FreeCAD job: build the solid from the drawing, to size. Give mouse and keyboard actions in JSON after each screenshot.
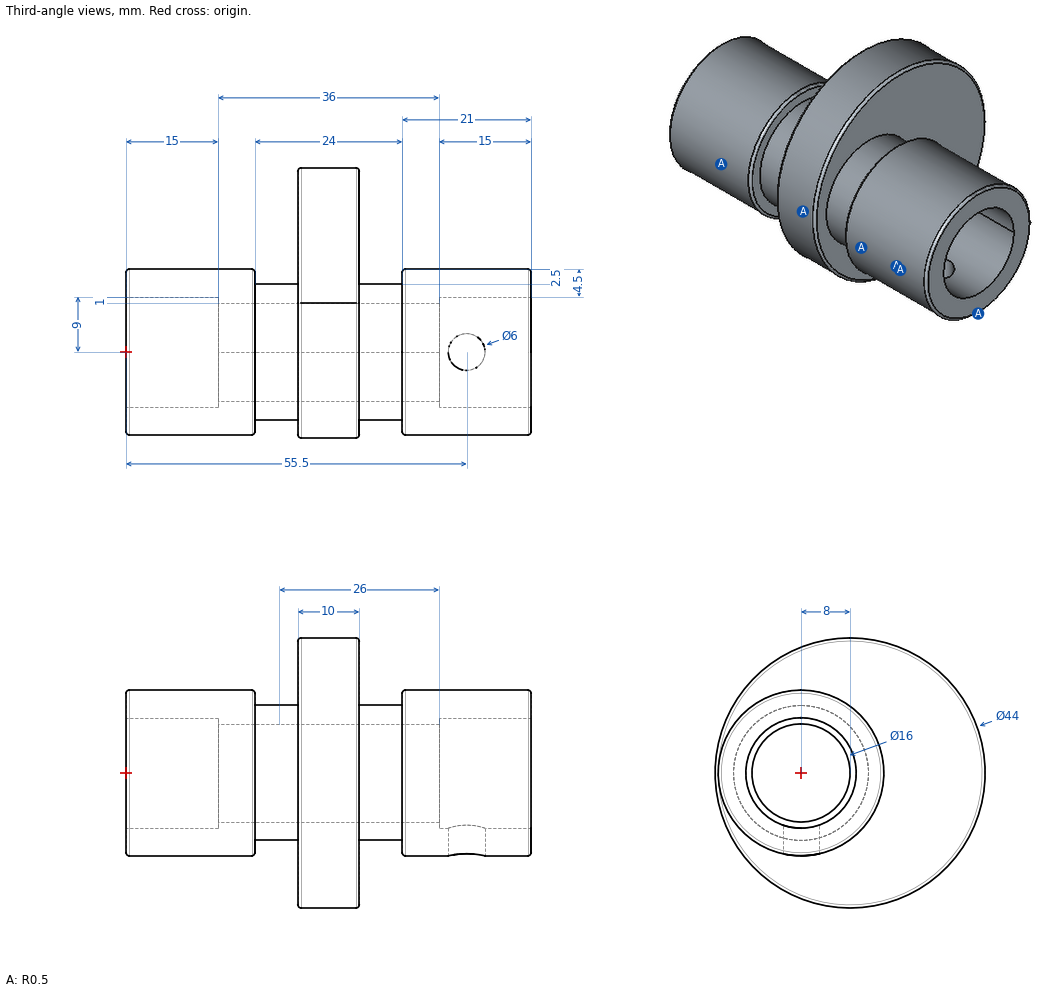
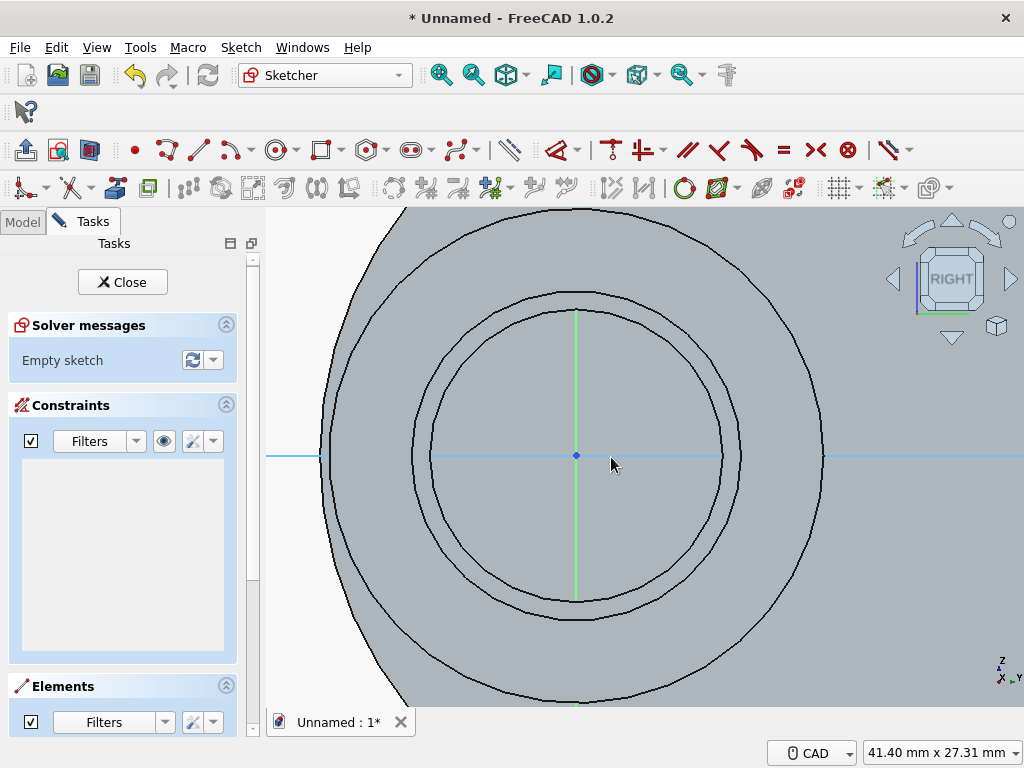
{"action": "left_click", "coordinate": [276, 150]}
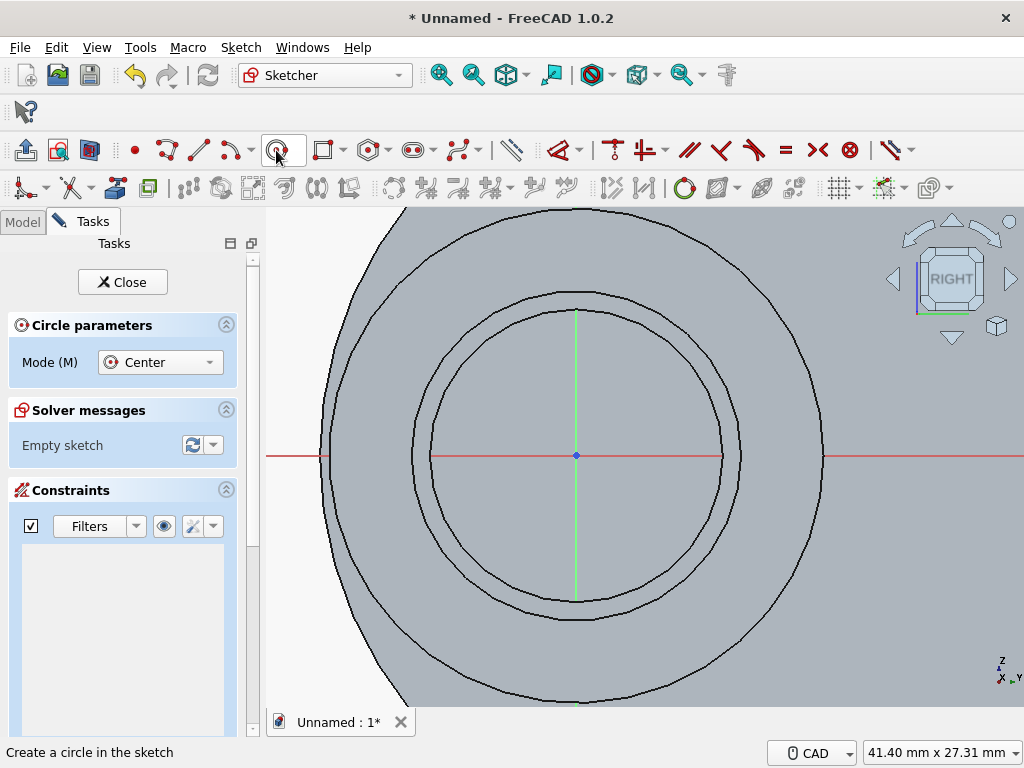
{"action": "left_click", "coordinate": [576, 456]}
{"action": "mouse_move", "coordinate": [680, 352]}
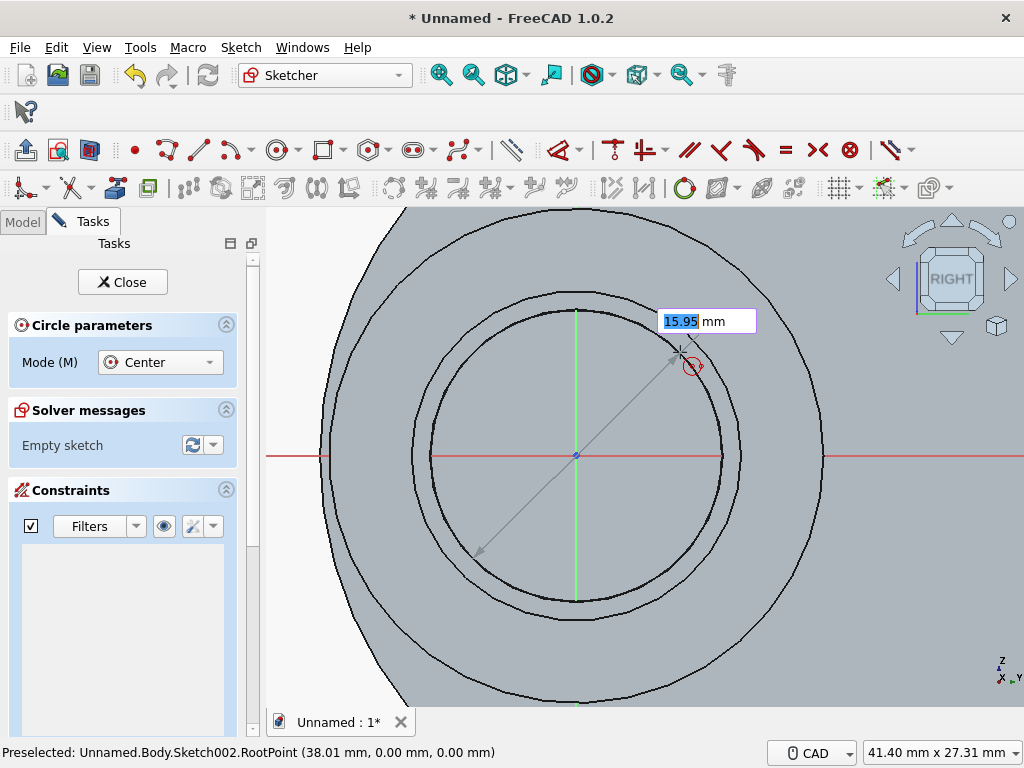
{"action": "type", "text": "16"}
{"action": "key", "text": "Return"}
{"action": "key", "text": "Escape"}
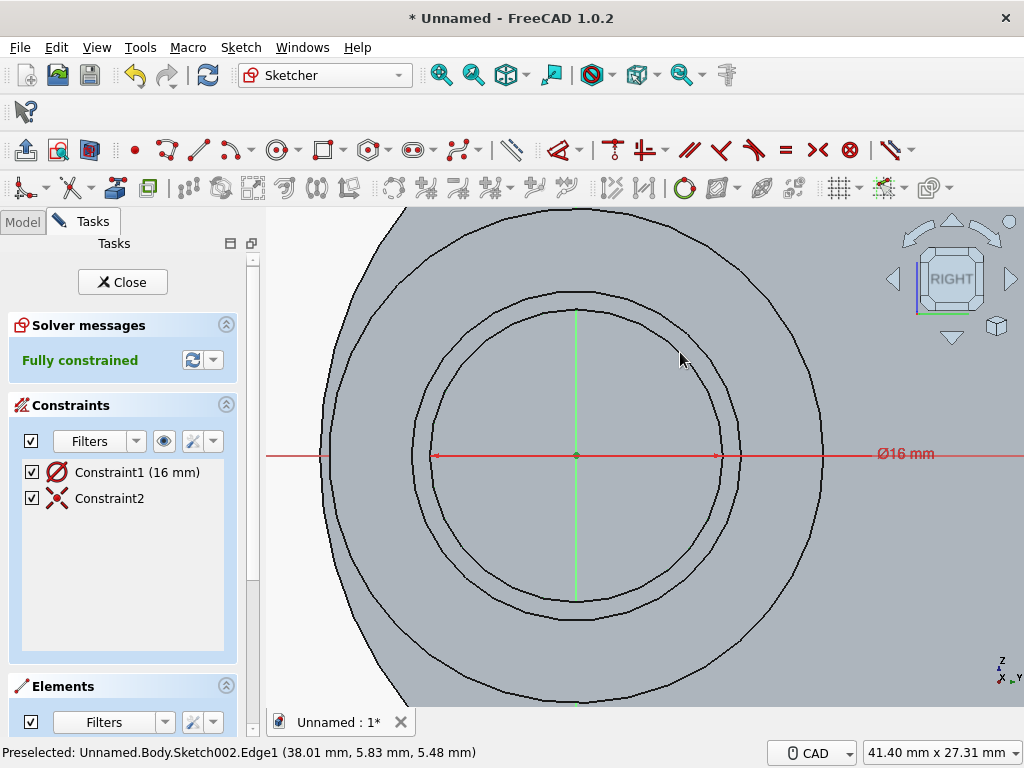
{"action": "left_click", "coordinate": [123, 282]}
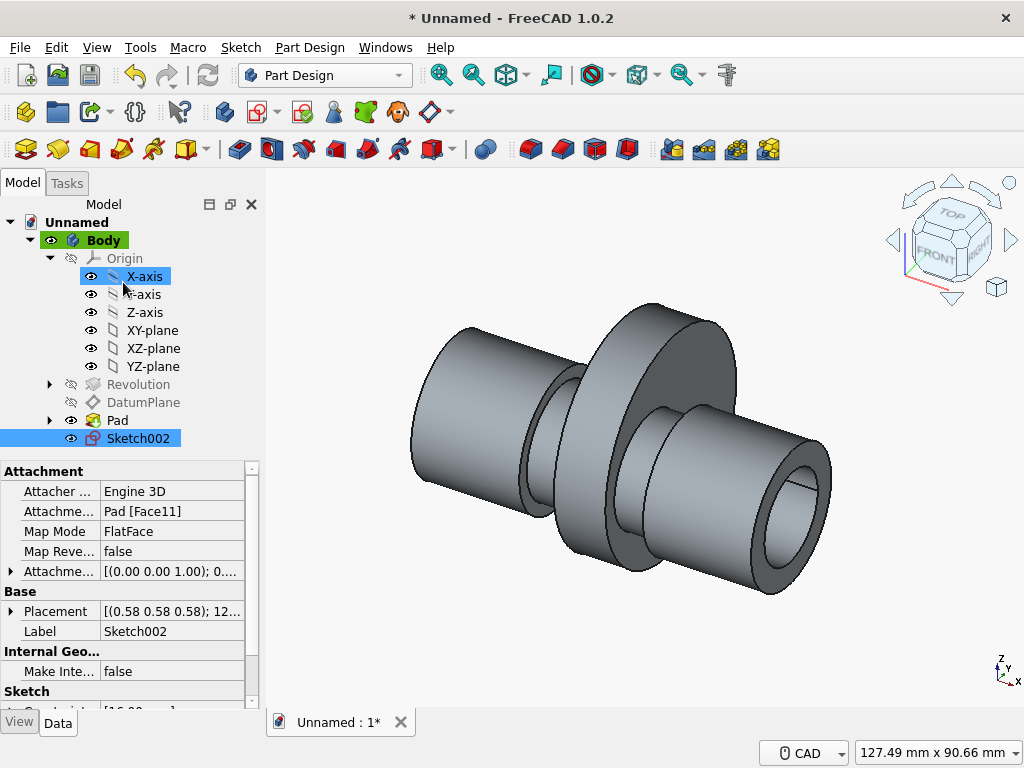
{"action": "left_click", "coordinate": [240, 150]}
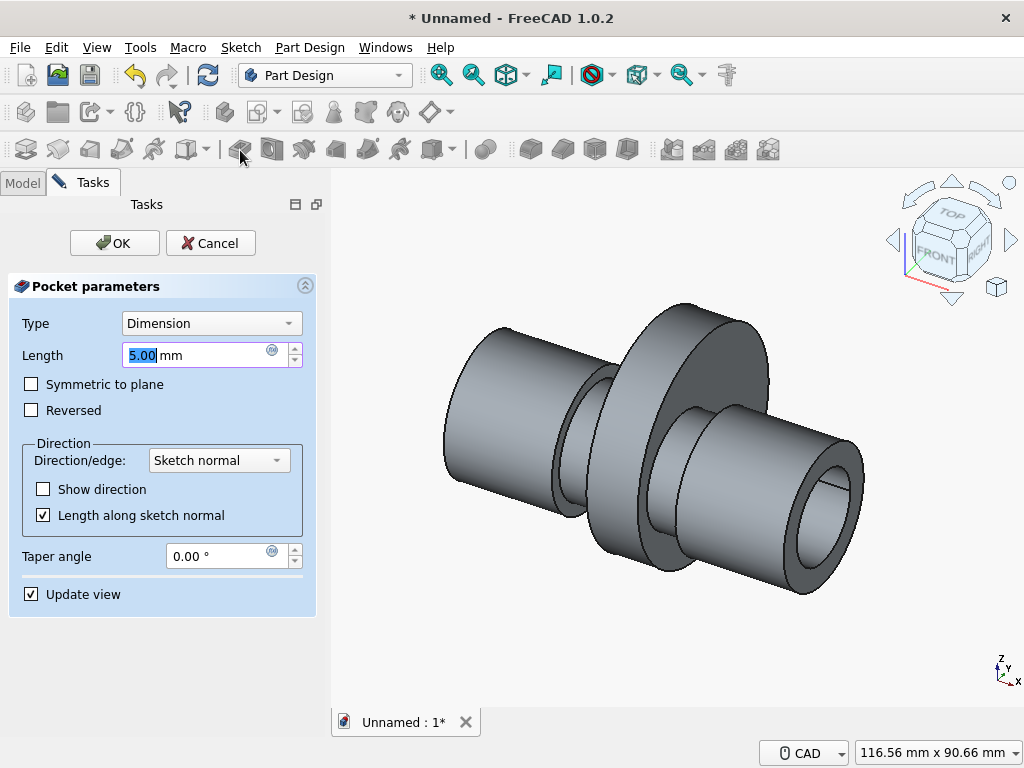
{"action": "type", "text": "26"}
{"action": "key", "text": "Tab"}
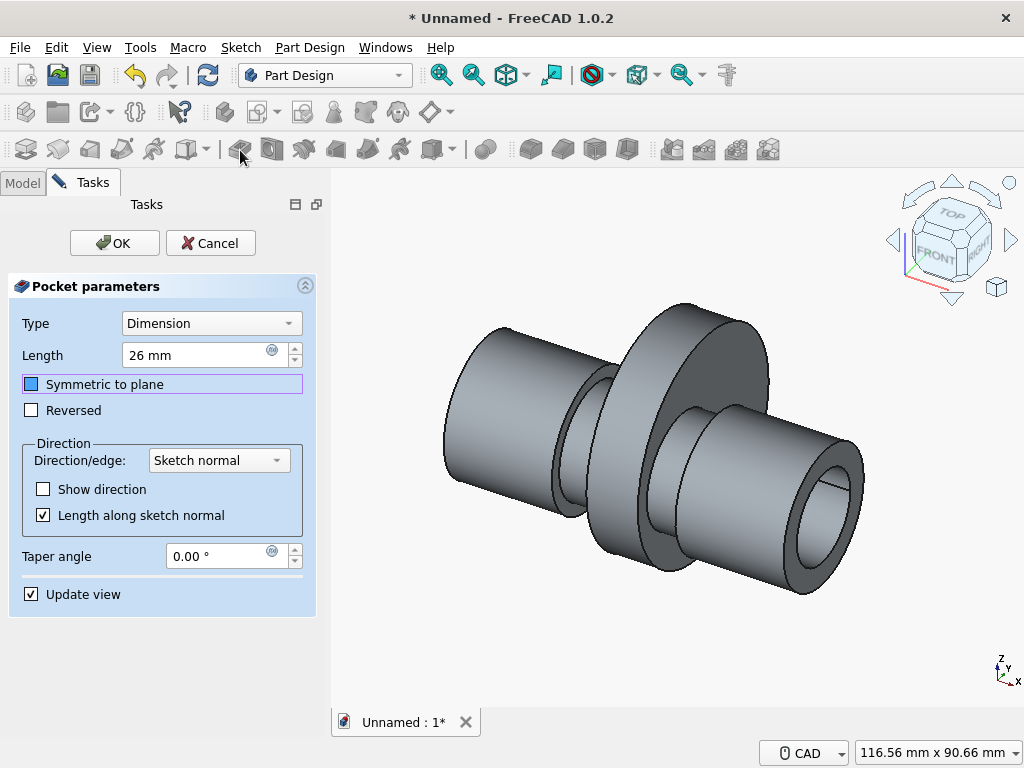
{"action": "left_click", "coordinate": [30, 384]}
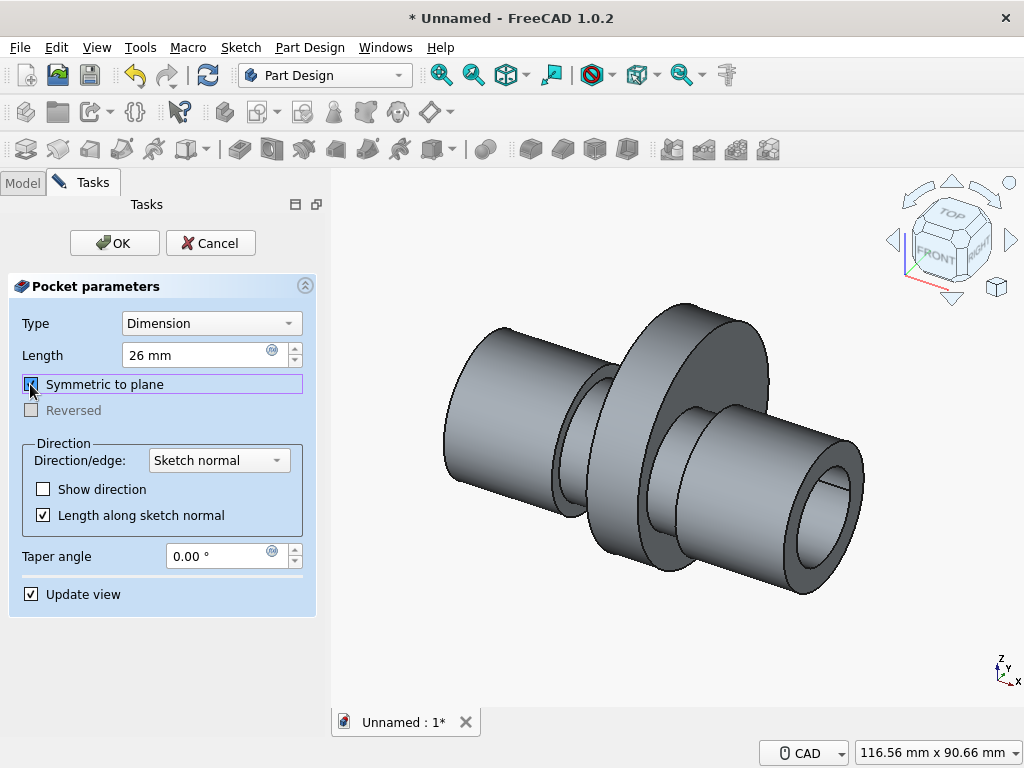
{"action": "left_click", "coordinate": [115, 243]}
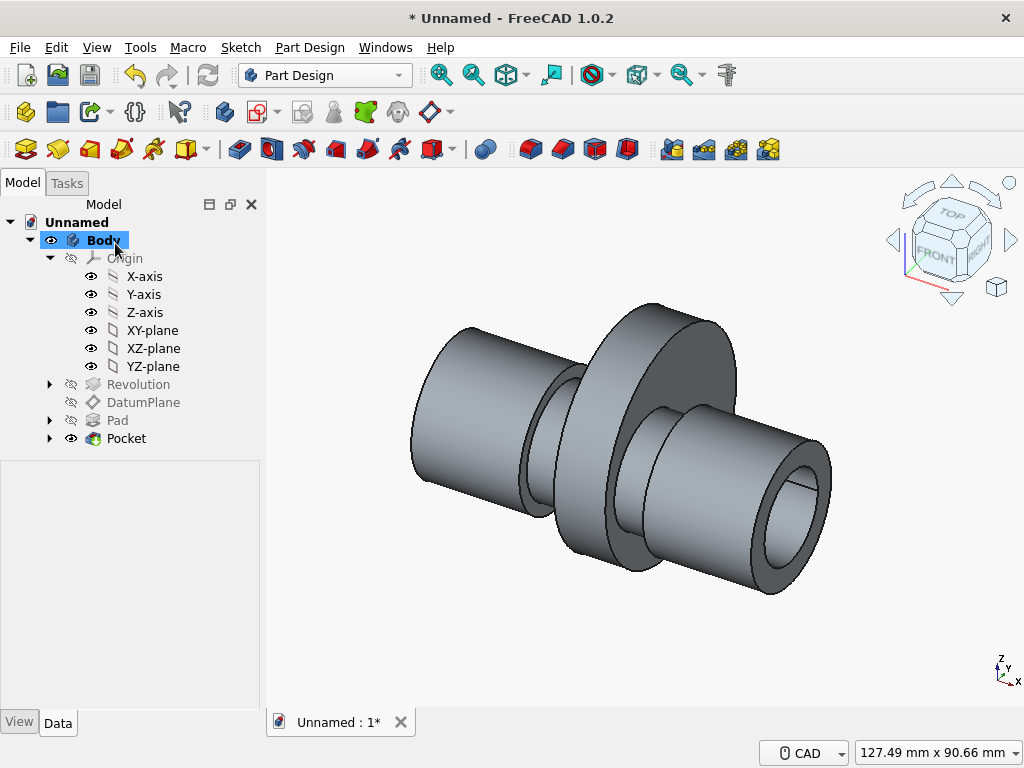
{"action": "left_click", "coordinate": [751, 556]}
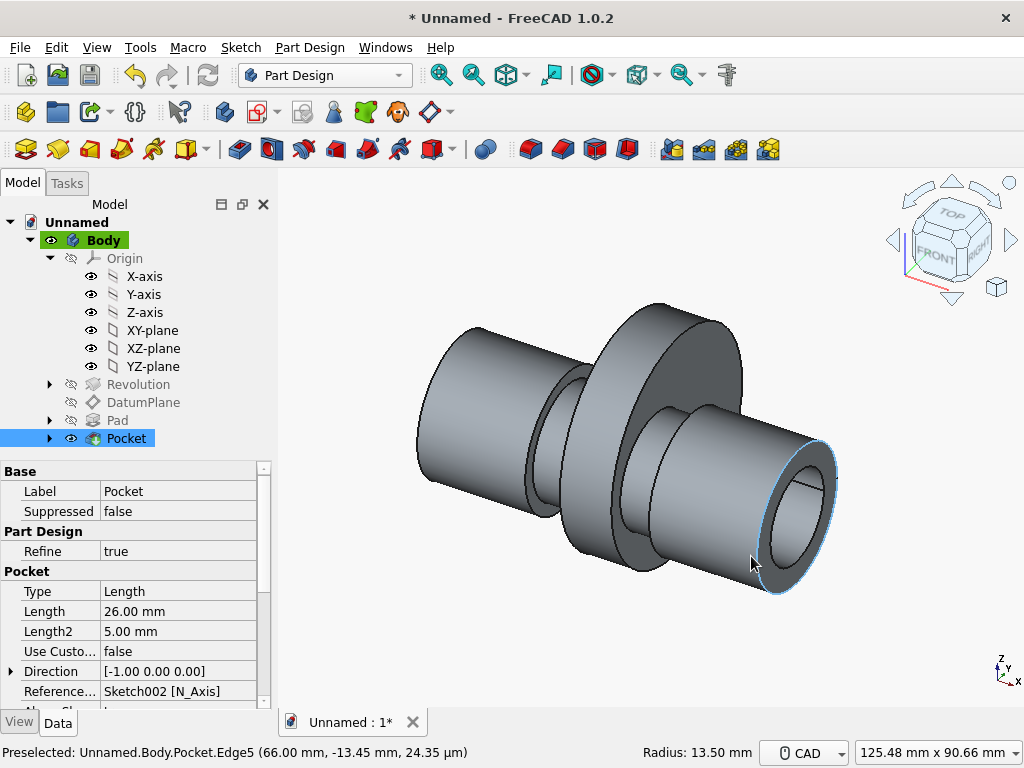
{"action": "left_click", "coordinate": [525, 480], "text": "ctrl"}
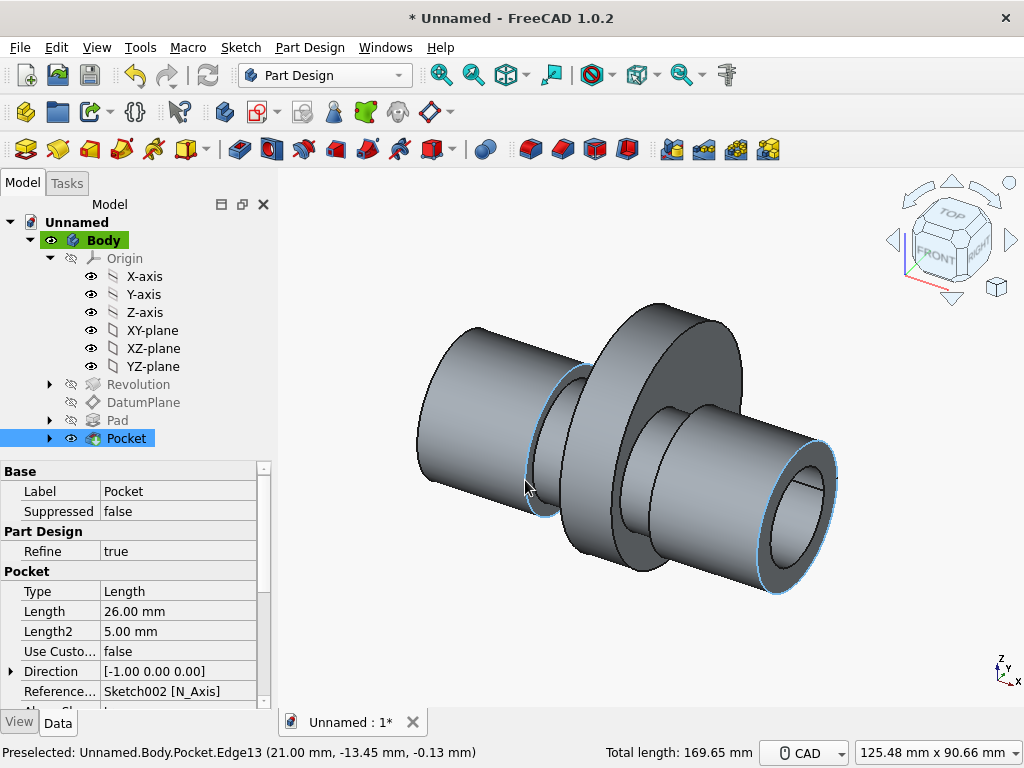
{"action": "left_click", "coordinate": [611, 510], "text": "ctrl"}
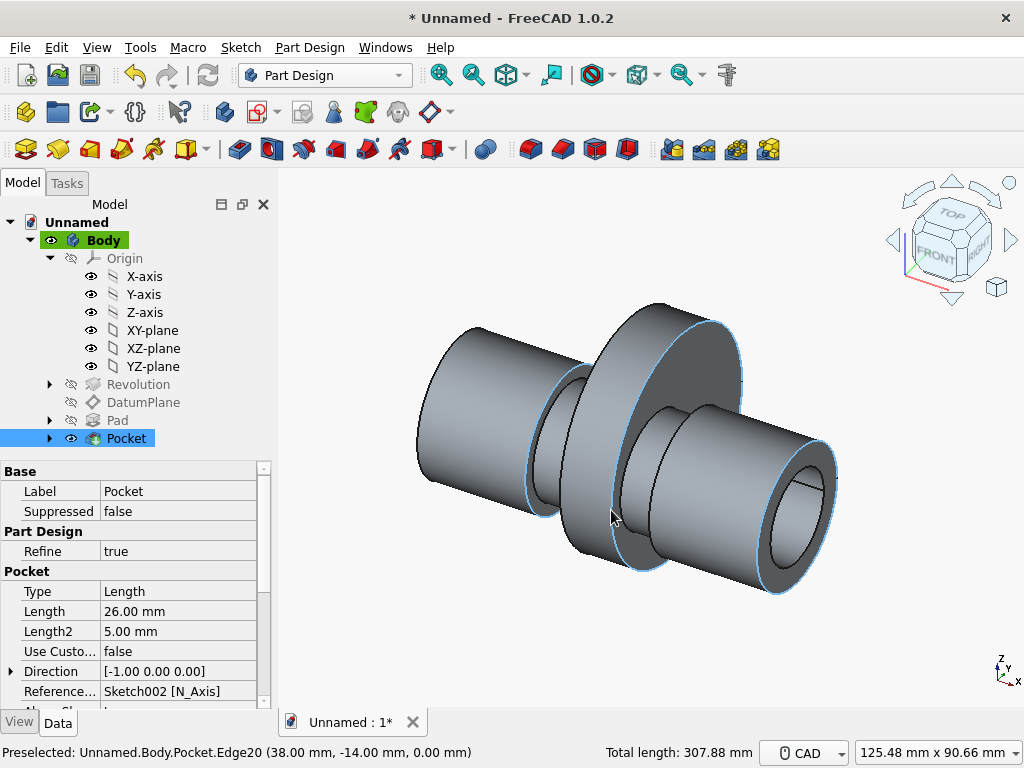
{"action": "key", "text": "0"}